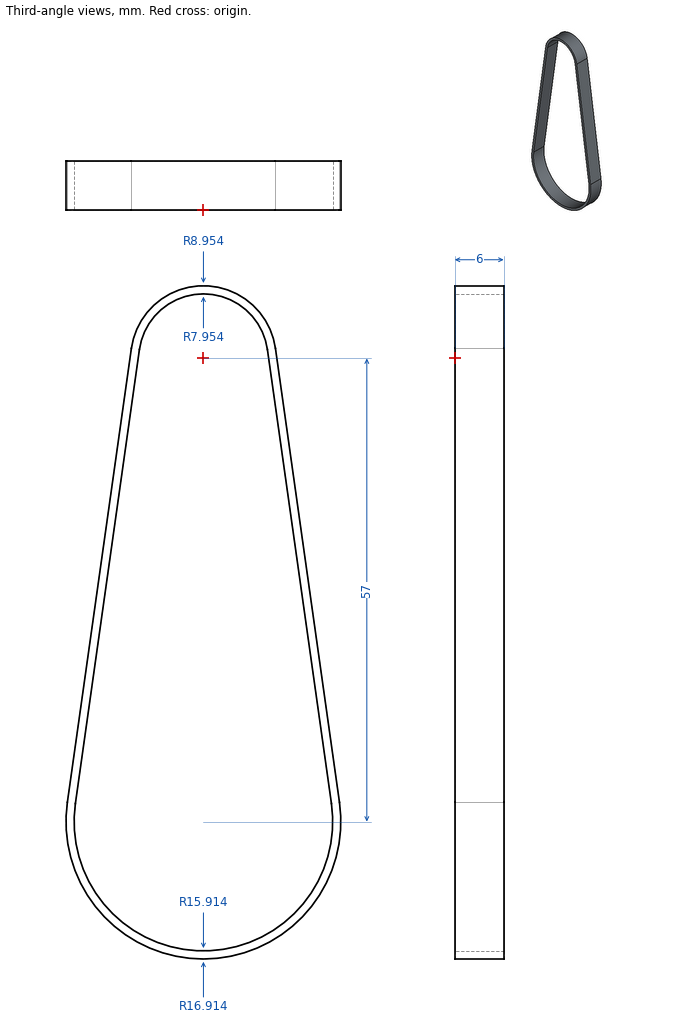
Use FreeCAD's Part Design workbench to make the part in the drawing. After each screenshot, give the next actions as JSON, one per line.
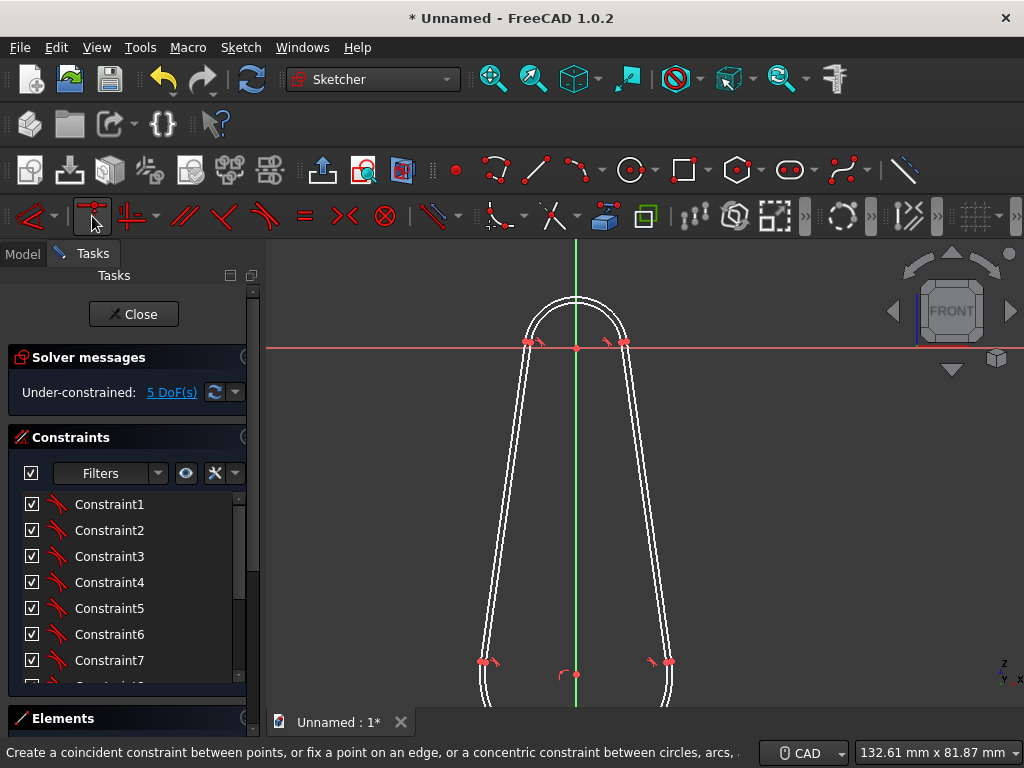
{"action": "left_click", "coordinate": [30, 216]}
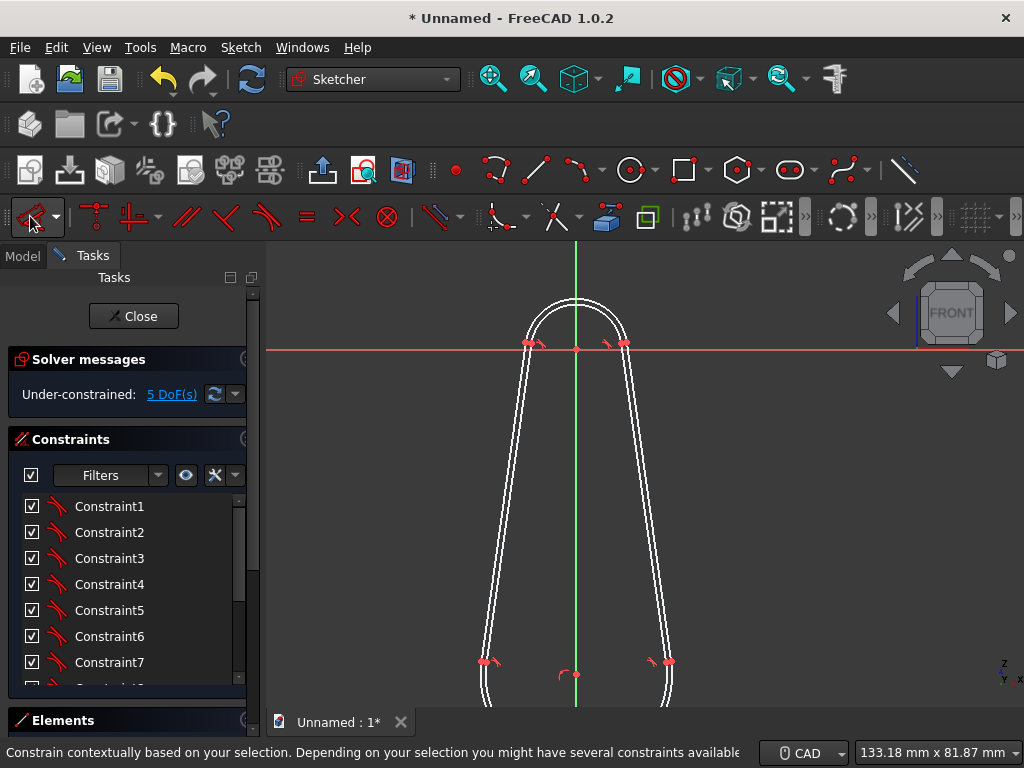
{"action": "scroll", "coordinate": [604, 307], "scroll_direction": "up", "scroll_amount": 5}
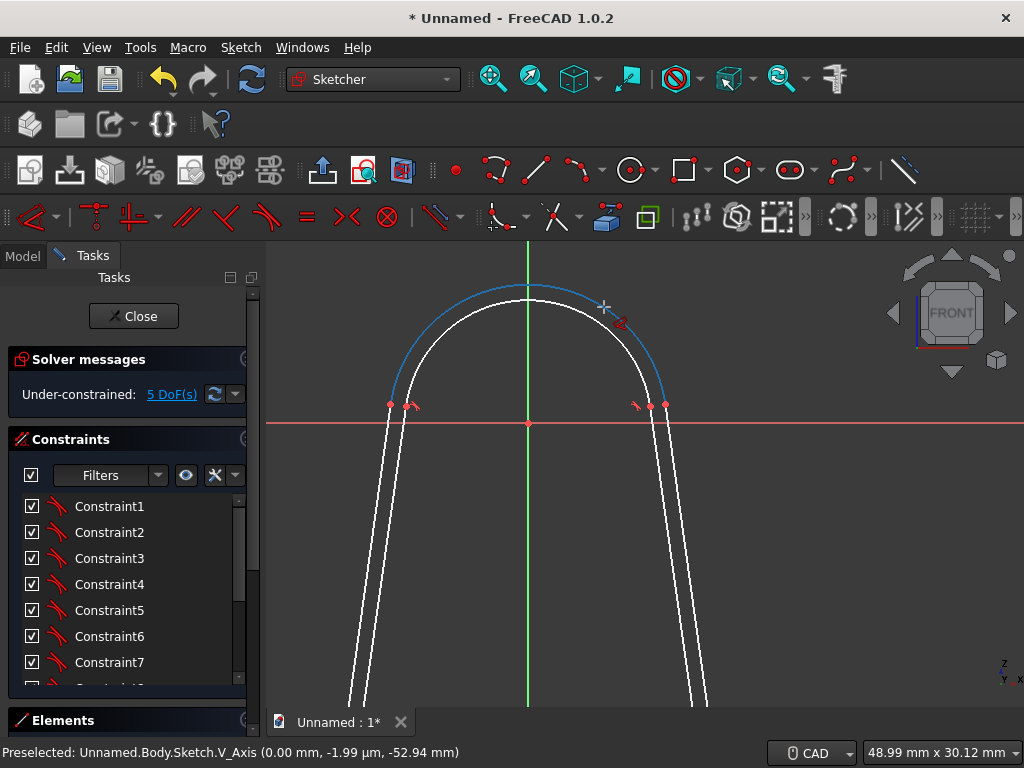
{"action": "left_click", "coordinate": [603, 307]}
{"action": "left_click", "coordinate": [620, 280]}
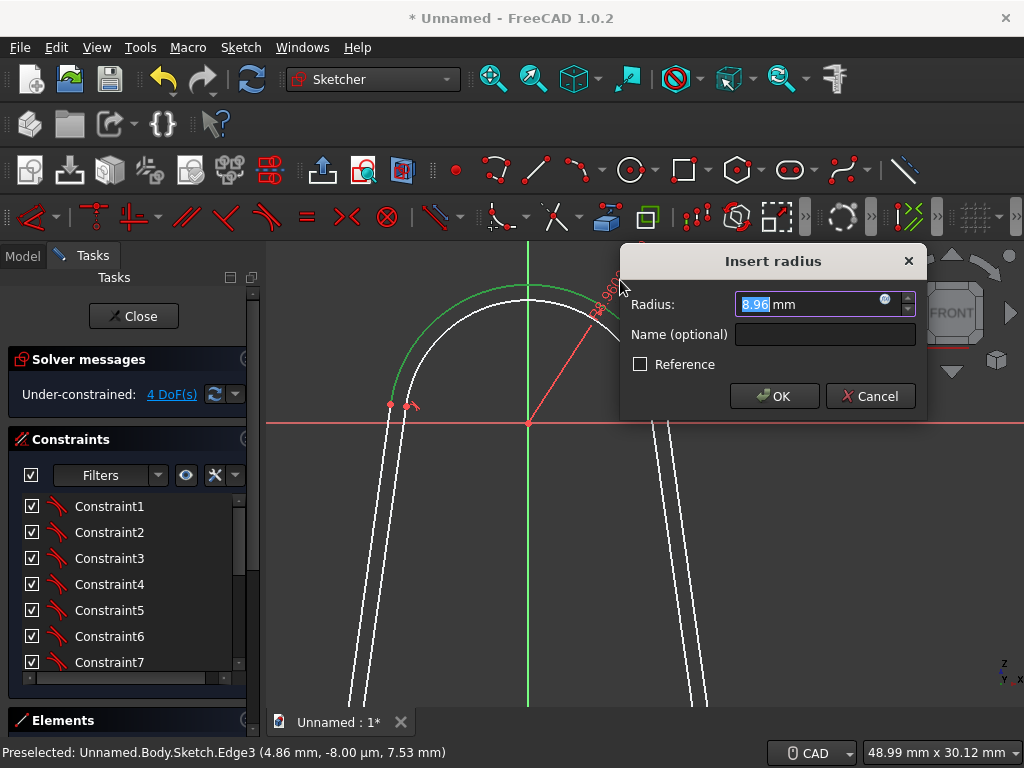
{"action": "type", "text": "8.954"}
{"action": "key", "text": "Return"}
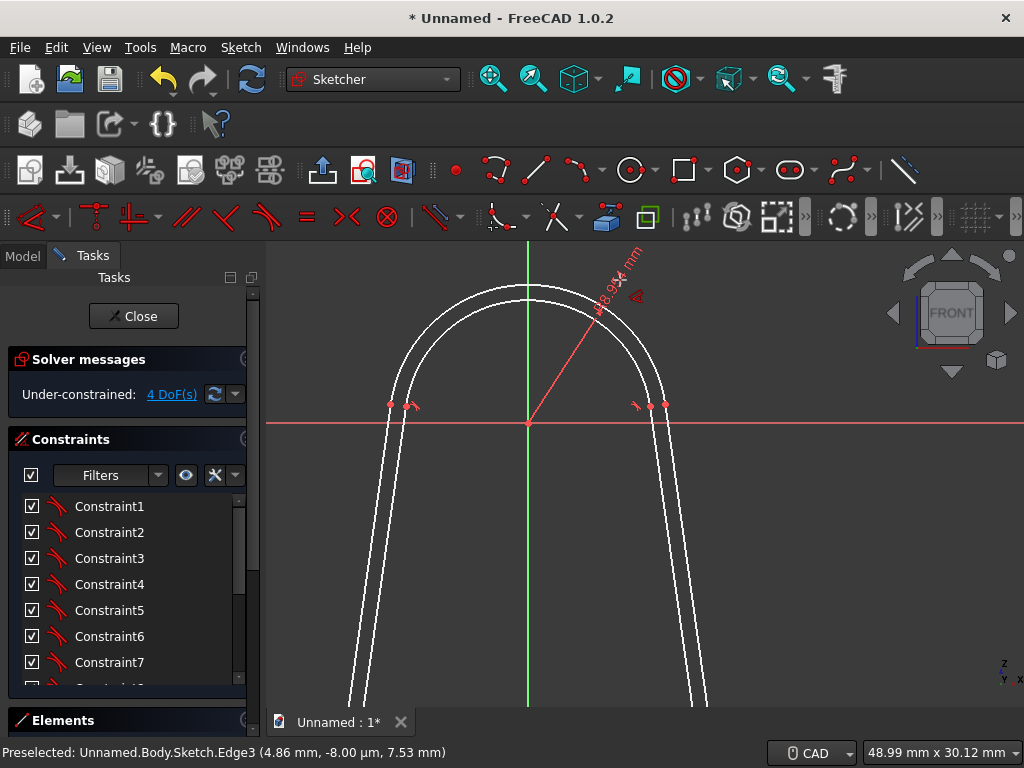
{"action": "scroll", "coordinate": [592, 326], "scroll_direction": "down", "scroll_amount": 7}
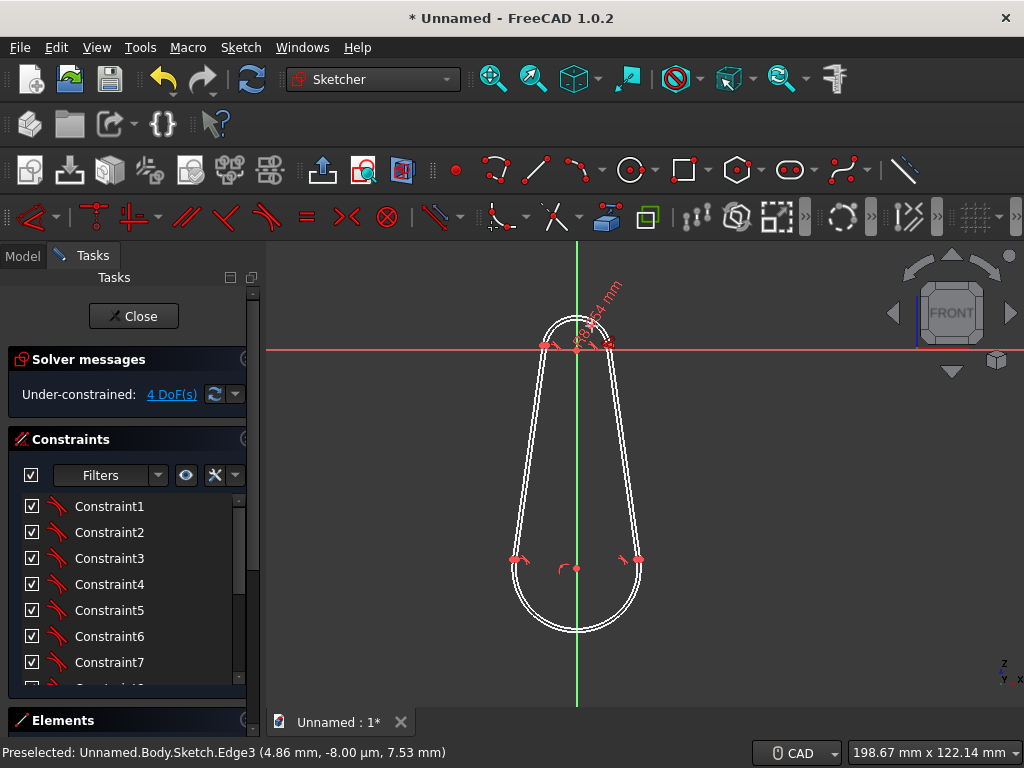
{"action": "scroll", "coordinate": [536, 618], "scroll_direction": "up", "scroll_amount": 7}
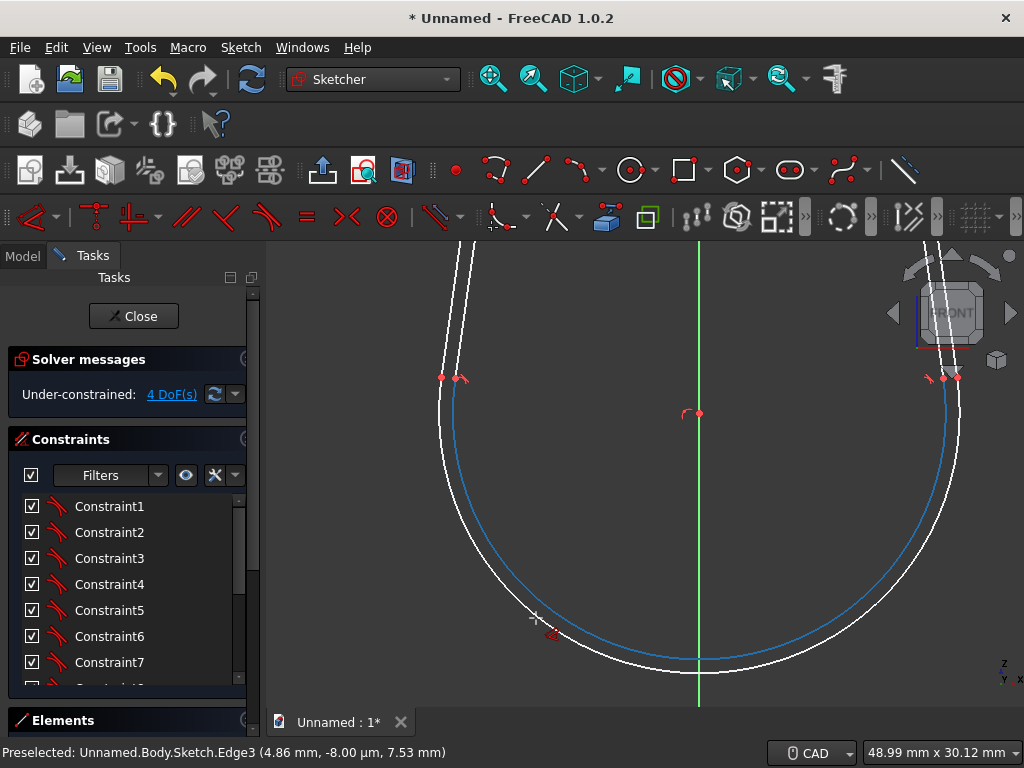
{"action": "left_click", "coordinate": [535, 615]}
{"action": "left_click", "coordinate": [515, 640]}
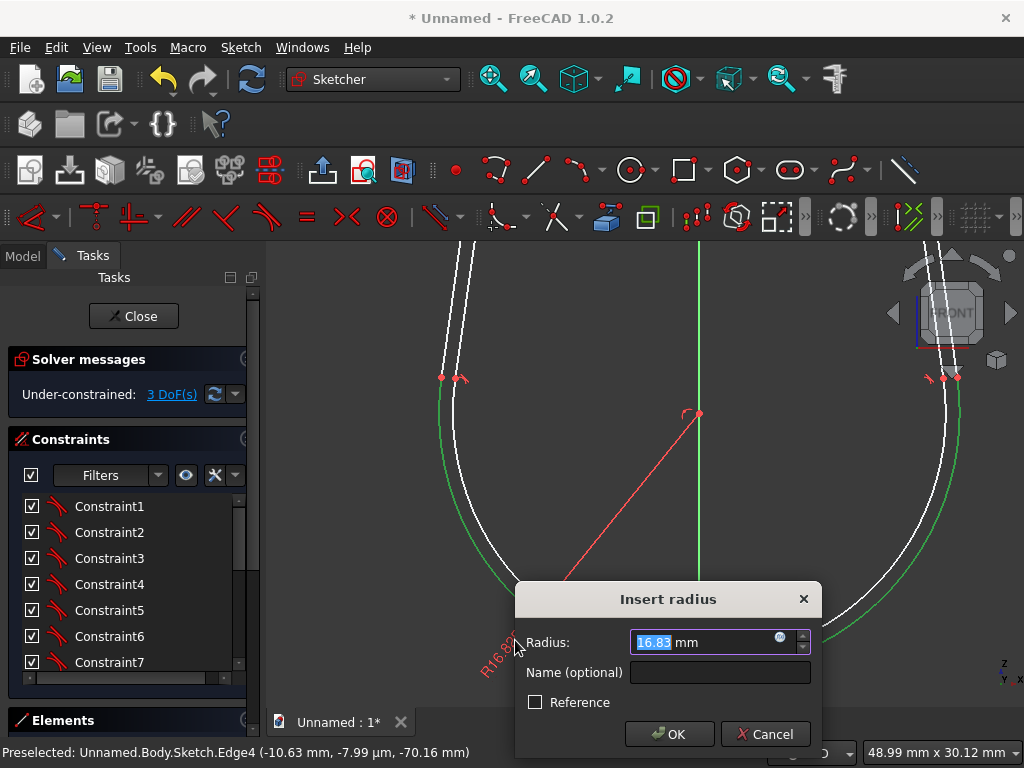
{"action": "type", "text": "16.914"}
{"action": "key", "text": "Return"}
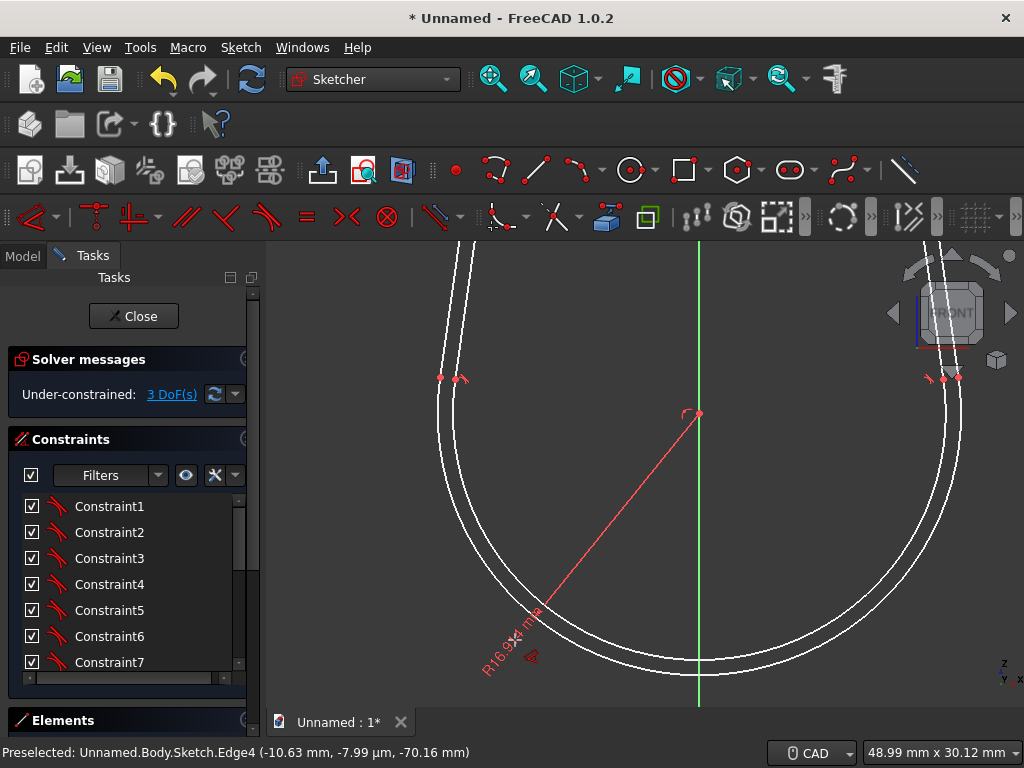
{"action": "left_click", "coordinate": [544, 605]}
{"action": "left_click", "coordinate": [442, 519]}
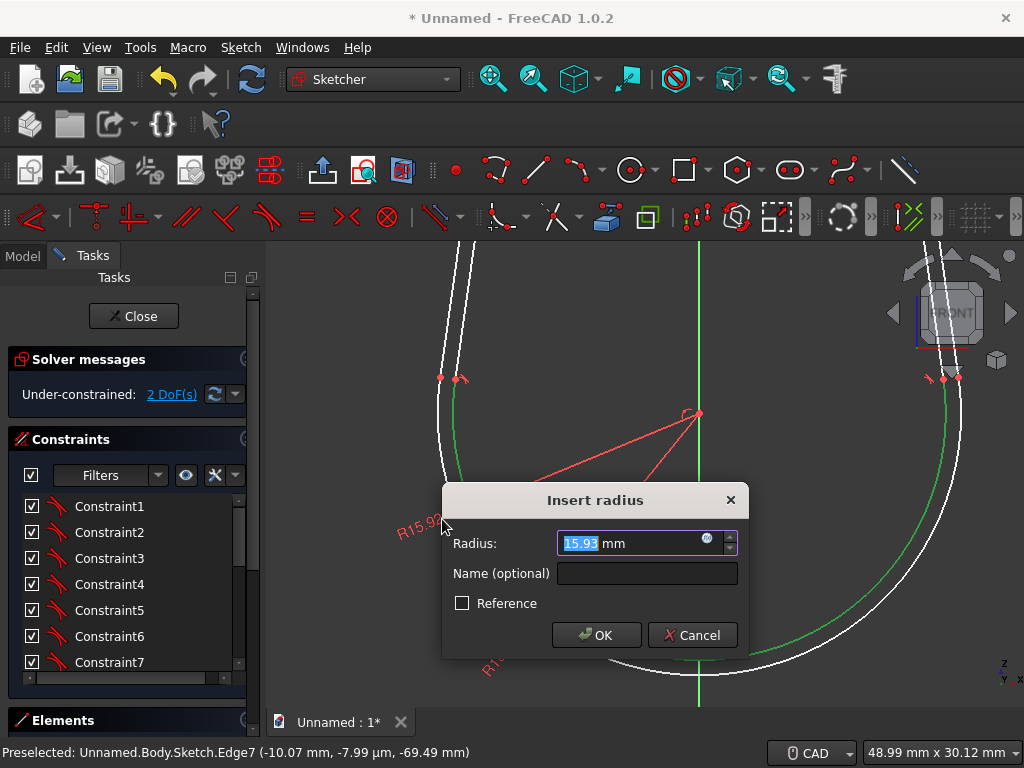
{"action": "type", "text": "15.914"}
{"action": "key", "text": "Return"}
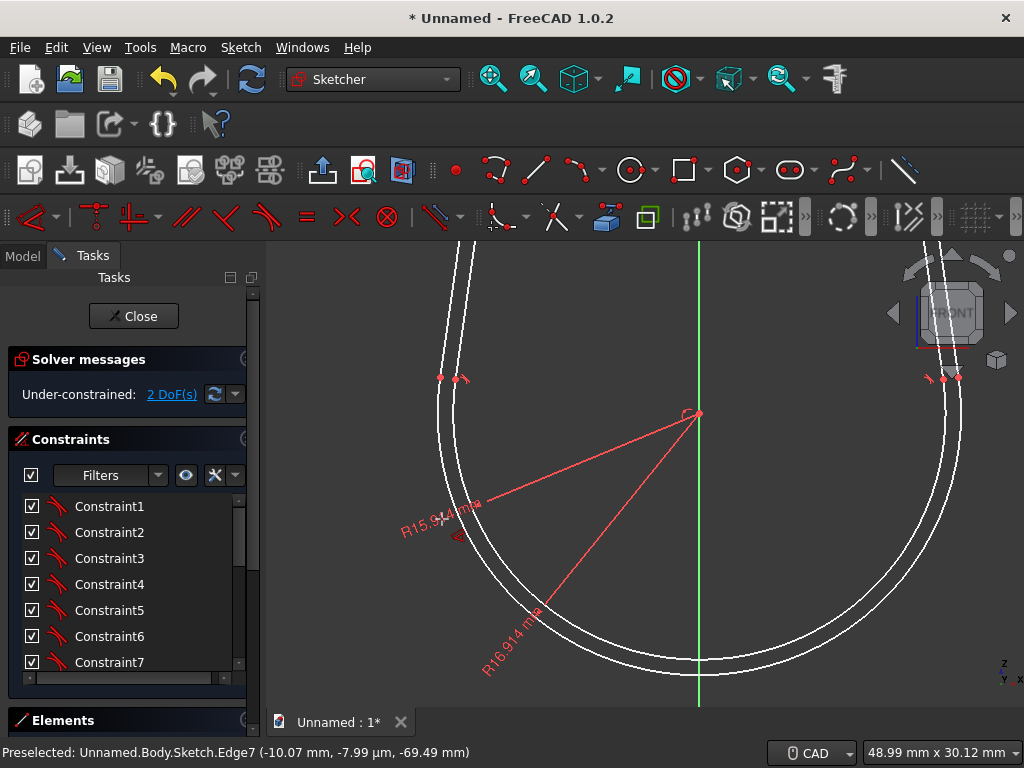
{"action": "scroll", "coordinate": [536, 619], "scroll_direction": "down", "scroll_amount": 7}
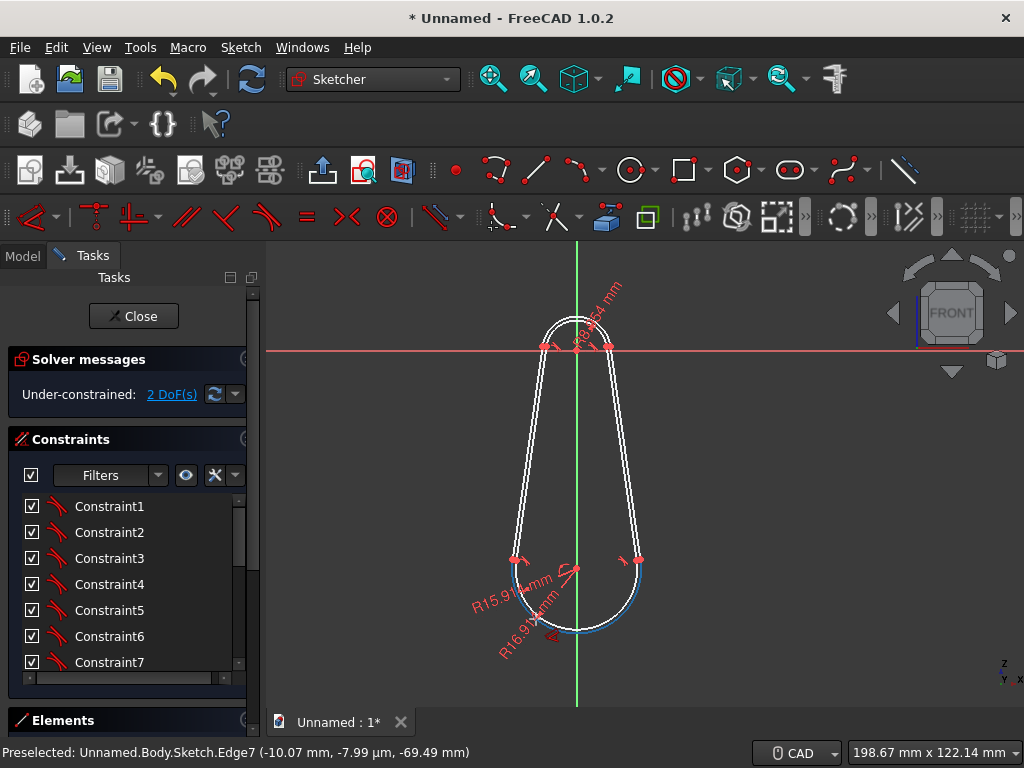
{"action": "scroll", "coordinate": [593, 325], "scroll_direction": "up", "scroll_amount": 7}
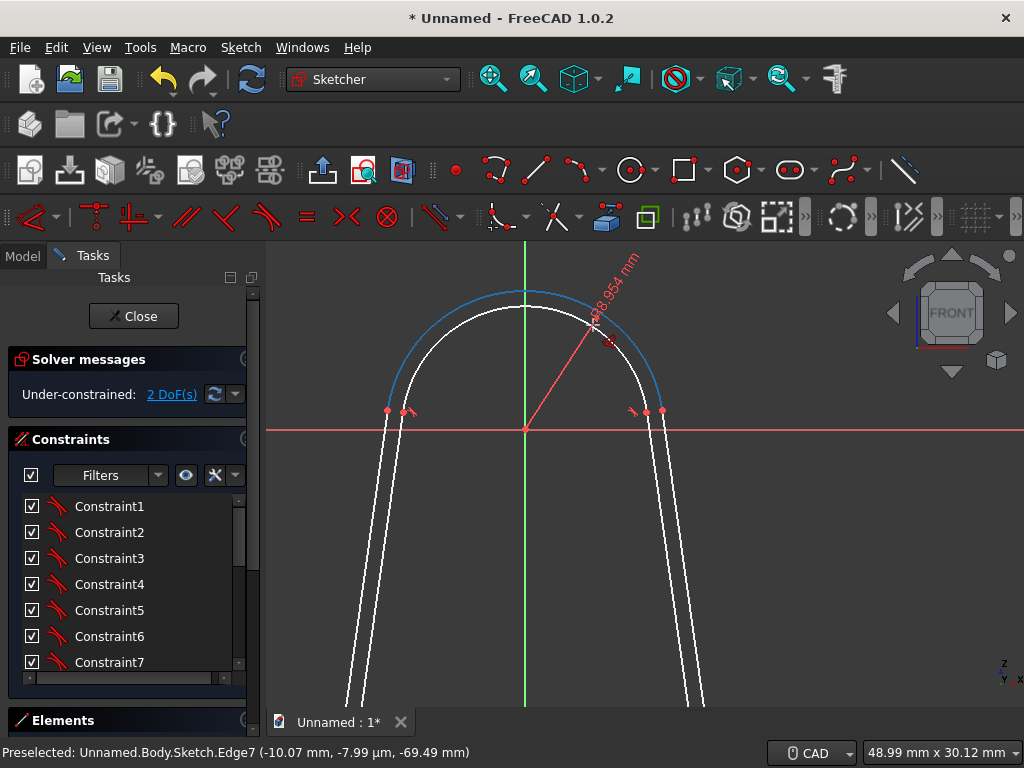
{"action": "left_click", "coordinate": [592, 326]}
{"action": "left_click", "coordinate": [662, 356]}